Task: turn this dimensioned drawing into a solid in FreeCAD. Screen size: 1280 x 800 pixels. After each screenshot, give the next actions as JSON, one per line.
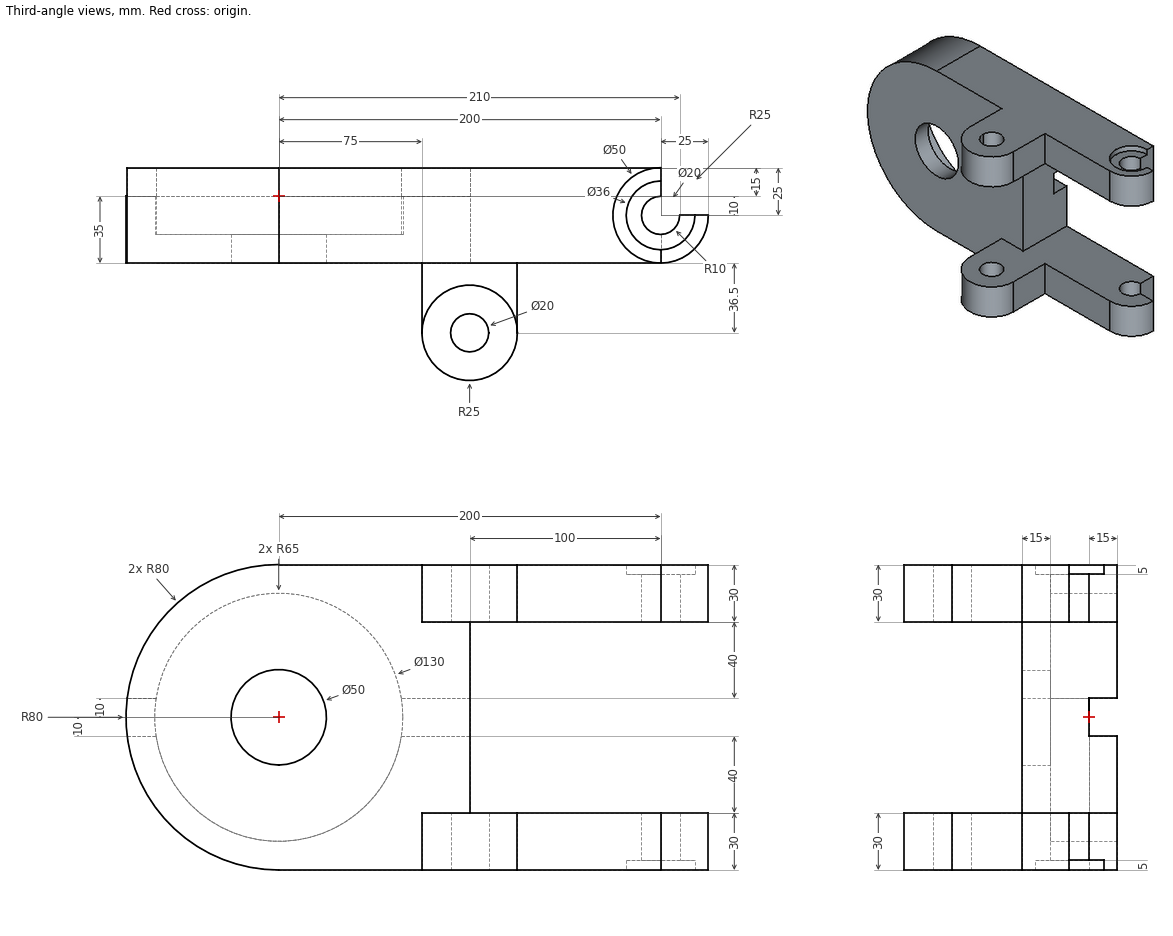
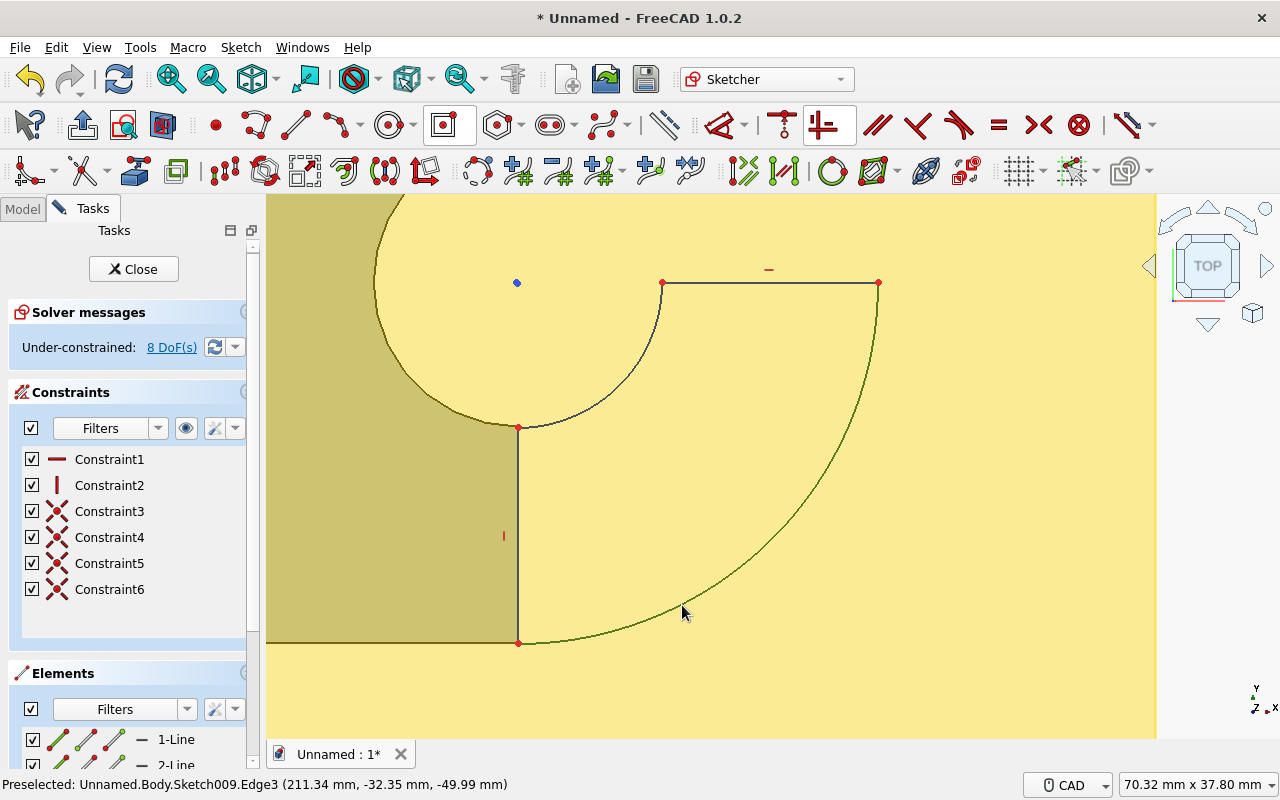
{"action": "left_click", "coordinate": [583, 412]}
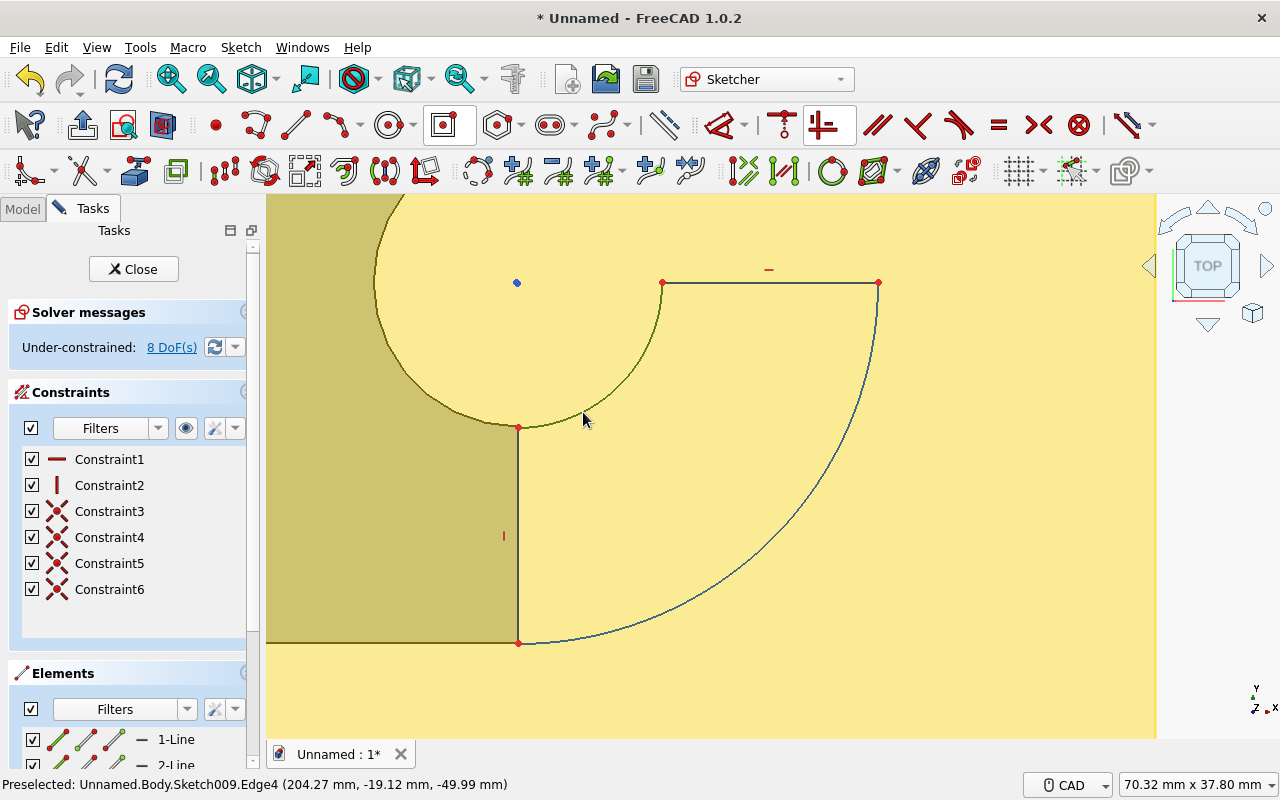
{"action": "key", "text": "c"}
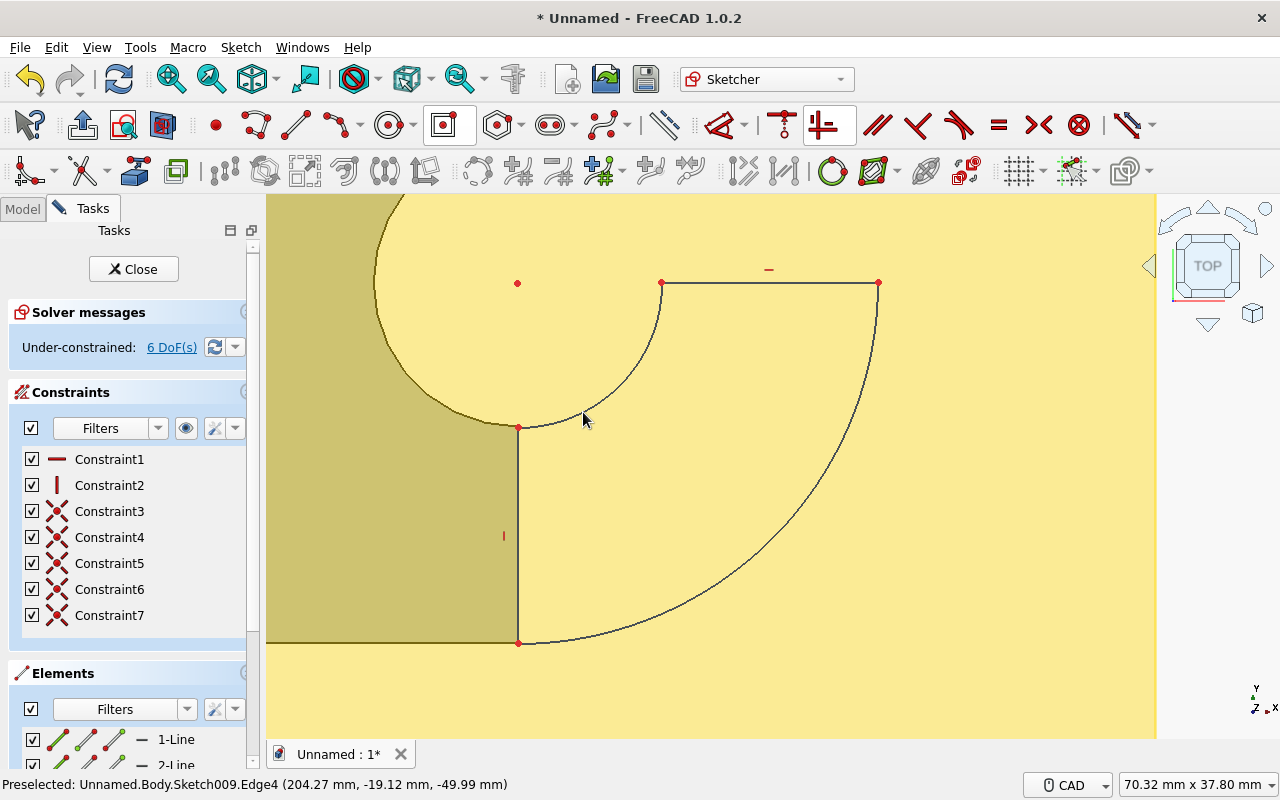
{"action": "key", "text": "d"}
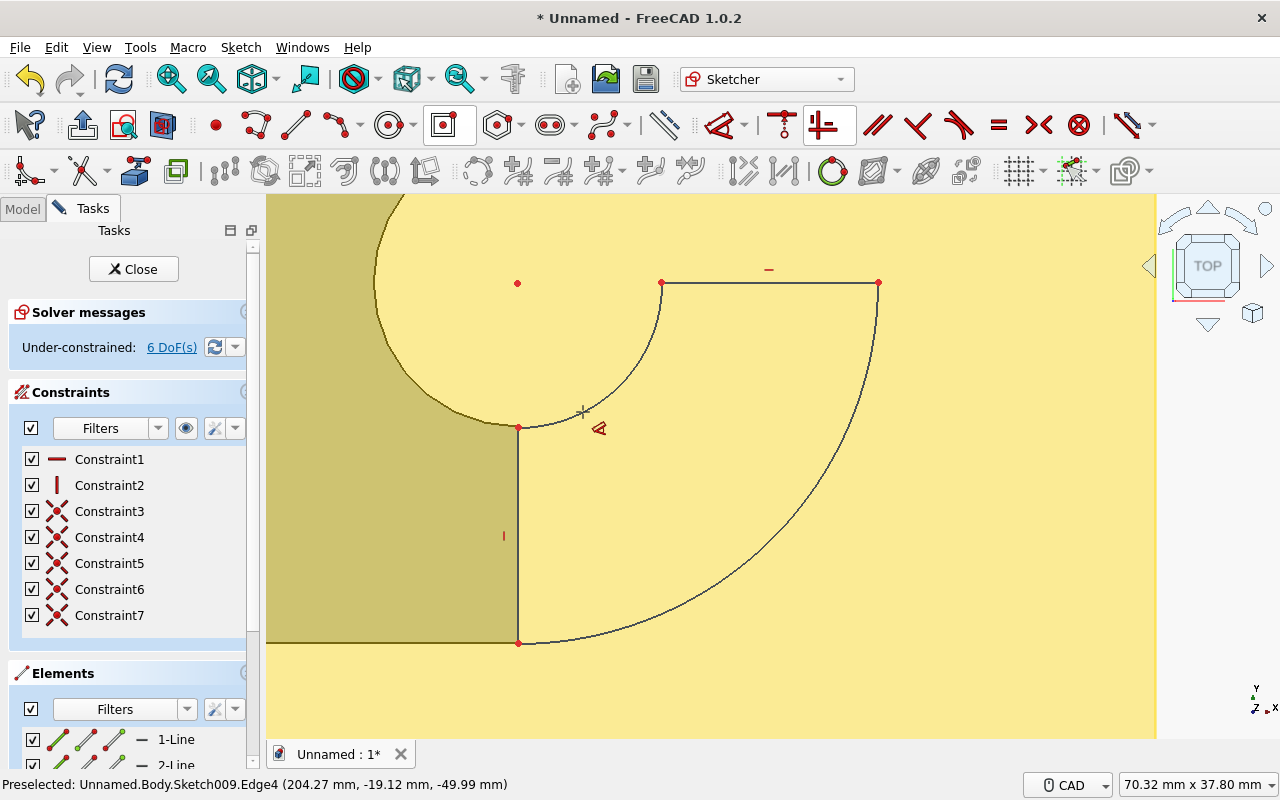
{"action": "left_click", "coordinate": [682, 605]}
{"action": "left_click", "coordinate": [697, 633]}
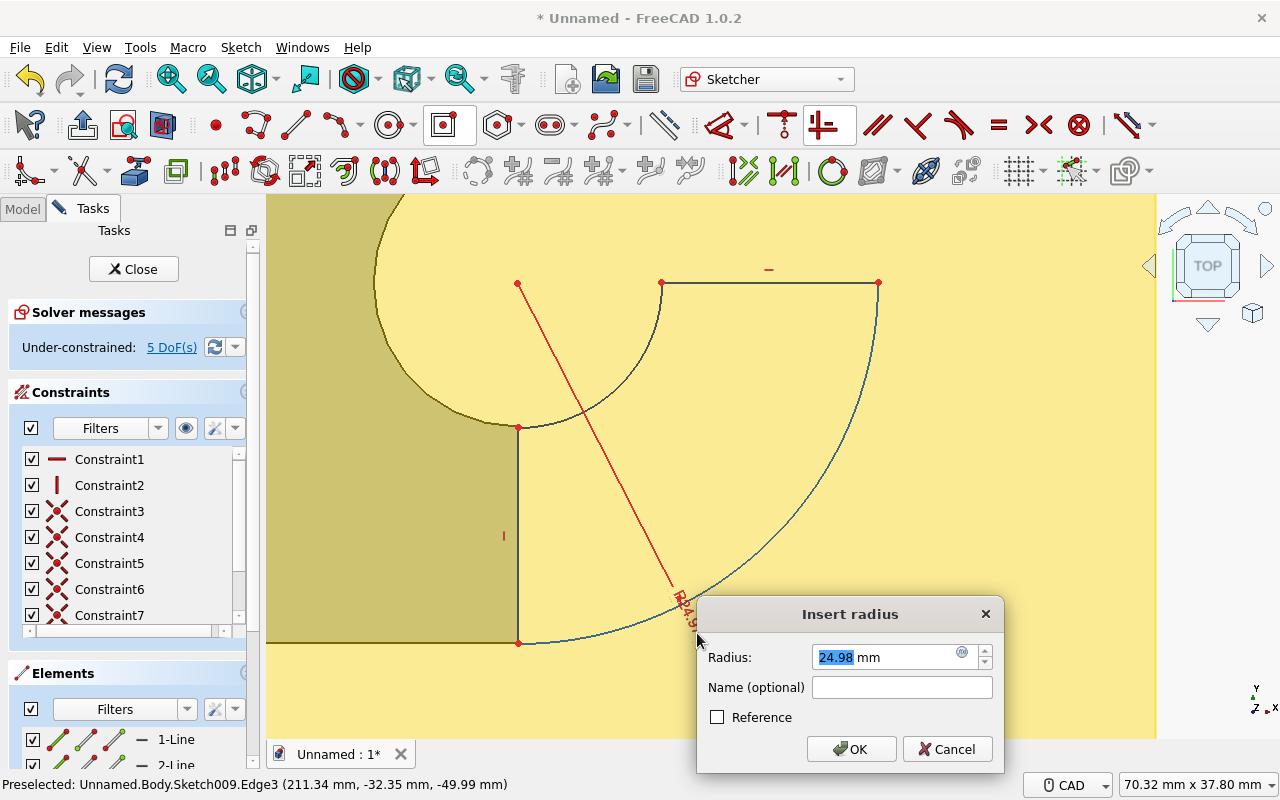
{"action": "type", "text": "25"}
{"action": "key", "text": "Return"}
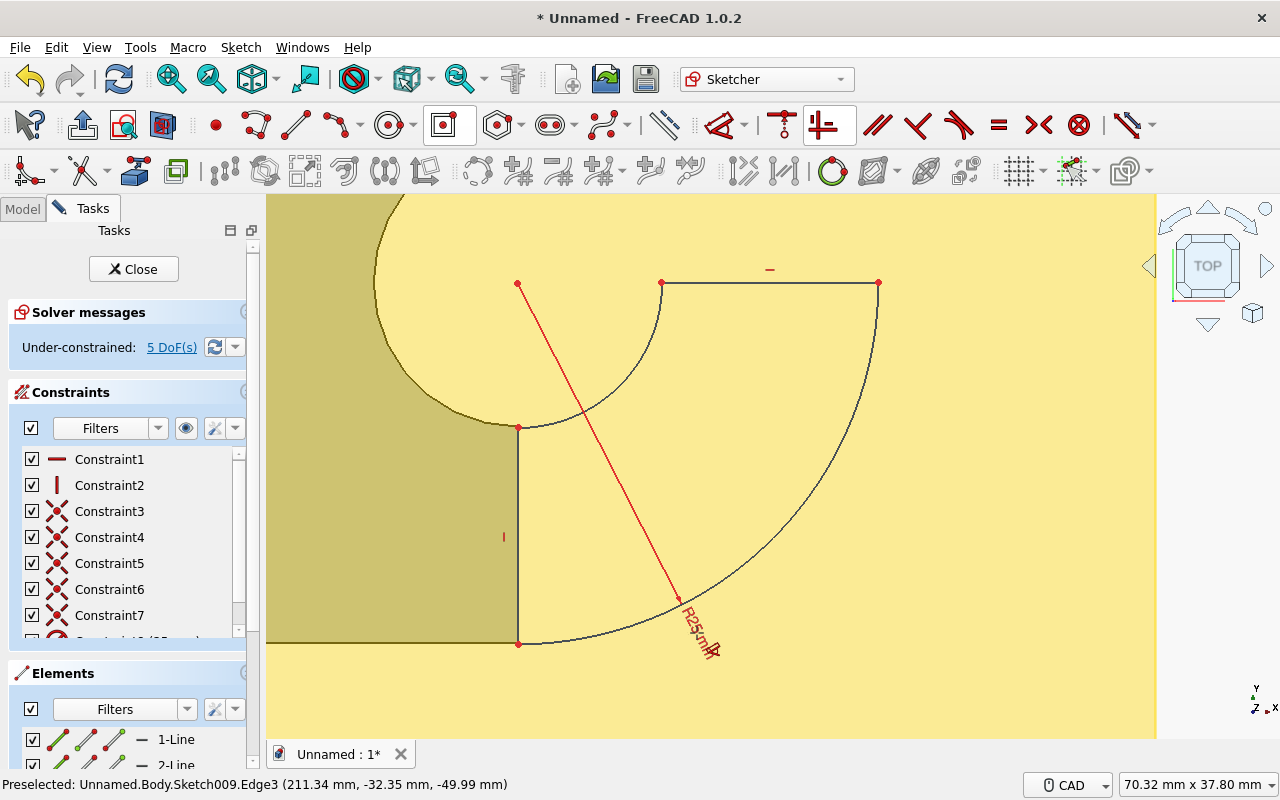
{"action": "left_click", "coordinate": [584, 412]}
{"action": "left_click", "coordinate": [599, 440]}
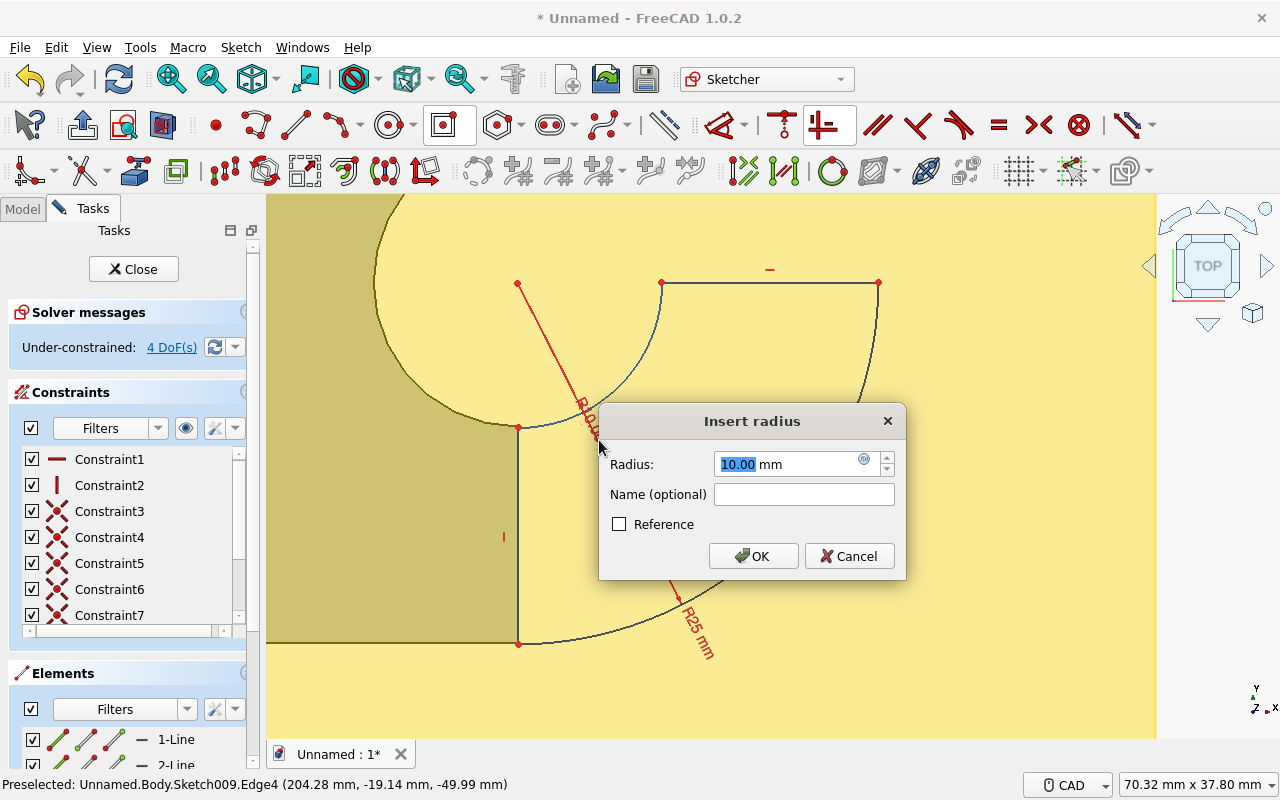
{"action": "type", "text": "10"}
{"action": "key", "text": "Return"}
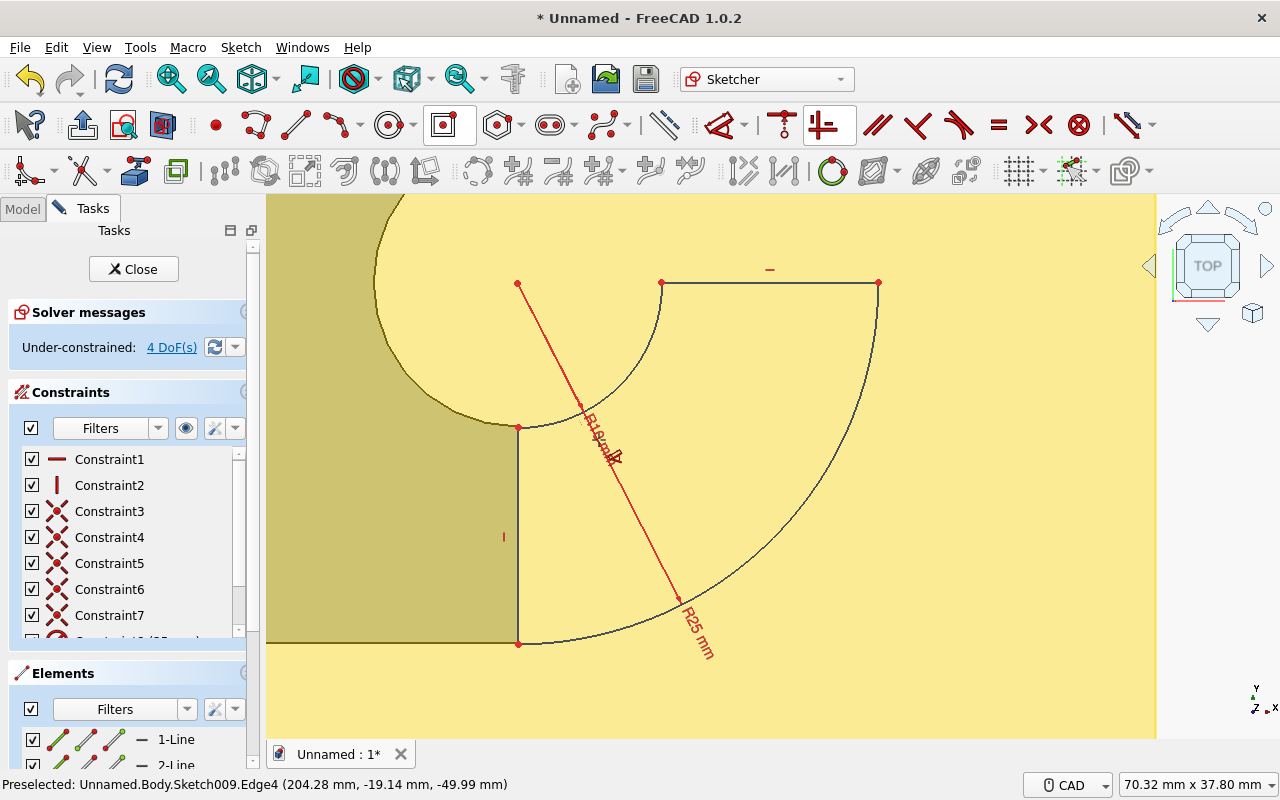
{"action": "left_click", "coordinate": [662, 283]}
{"action": "left_click", "coordinate": [696, 252]}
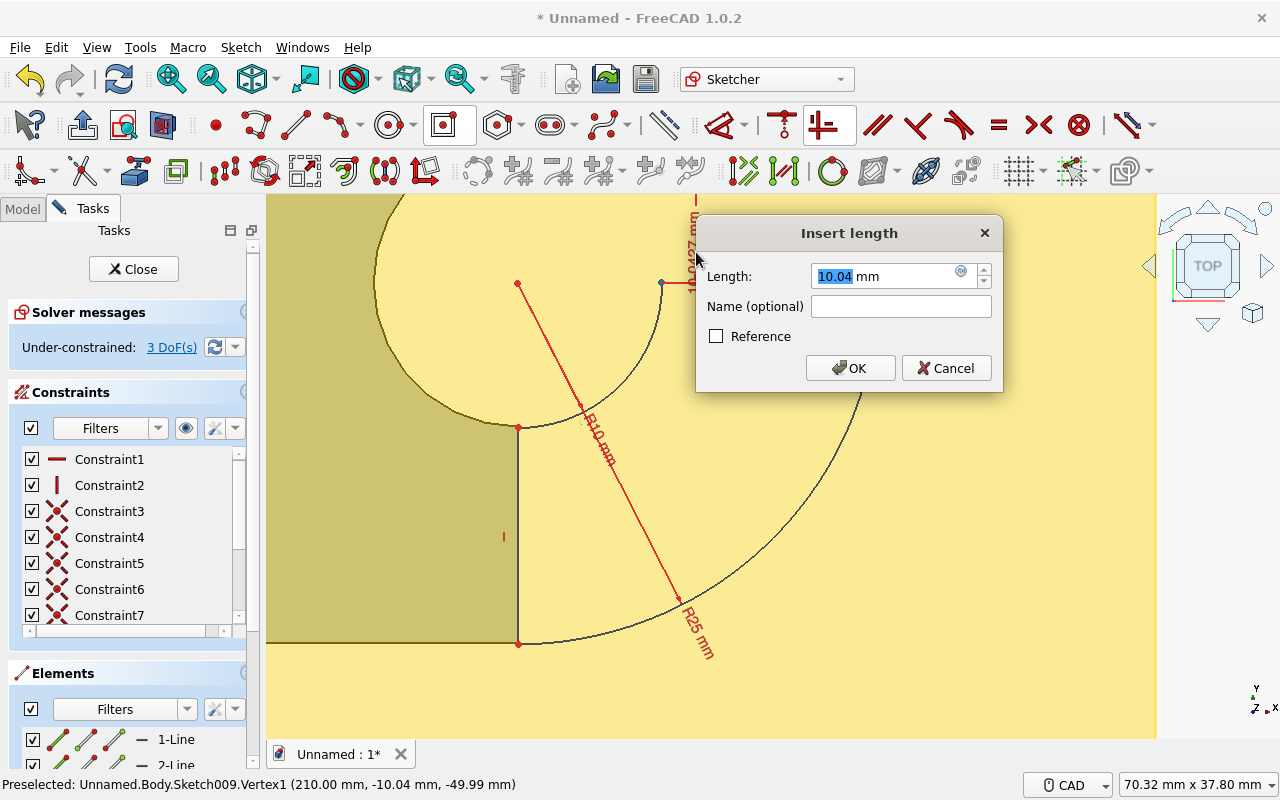
{"action": "type", "text": "10"}
{"action": "key", "text": "Return"}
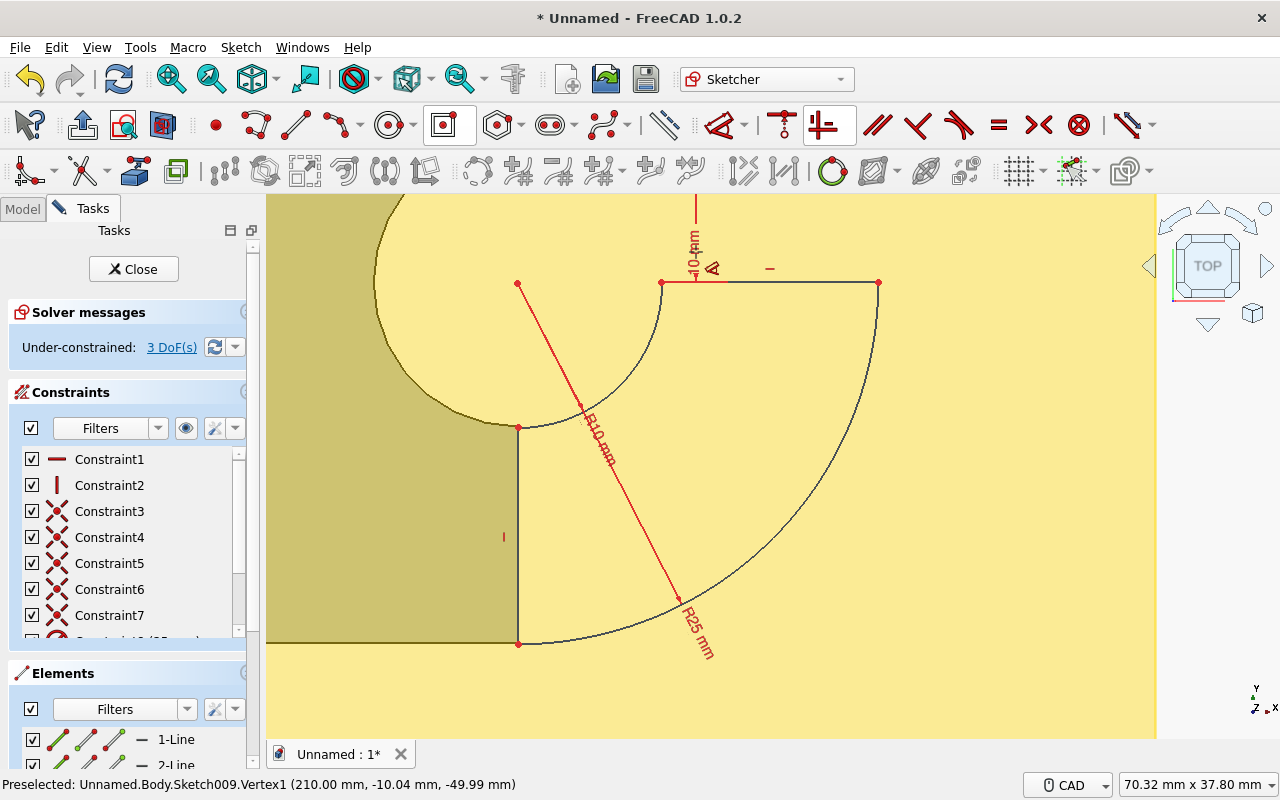
{"action": "left_click", "coordinate": [518, 644]}
{"action": "left_click", "coordinate": [552, 336]}